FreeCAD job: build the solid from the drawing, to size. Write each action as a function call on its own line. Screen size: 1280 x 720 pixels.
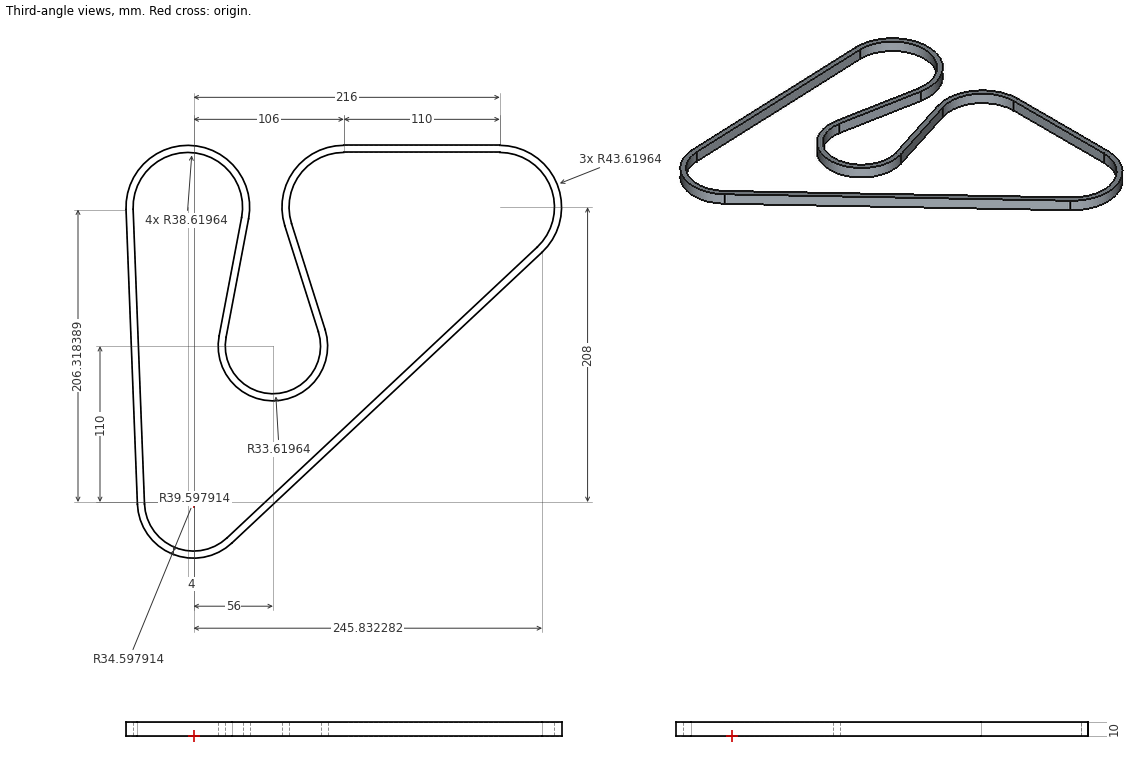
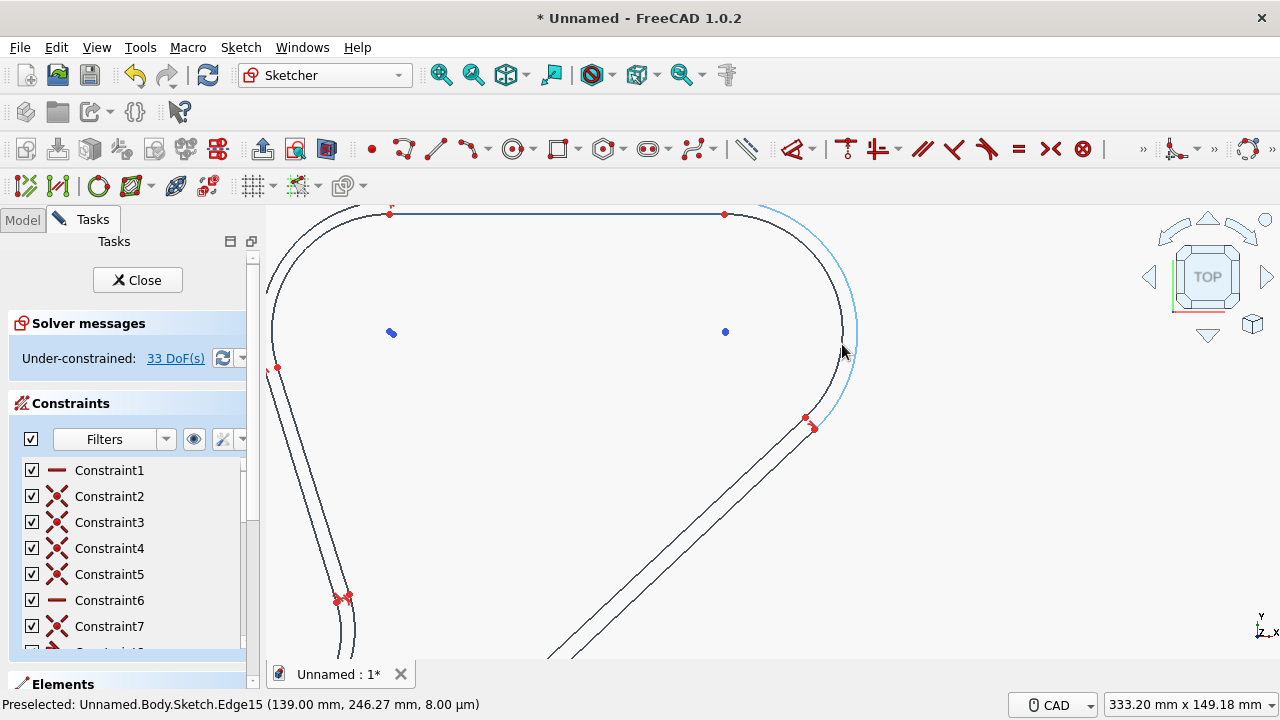
click(842, 343)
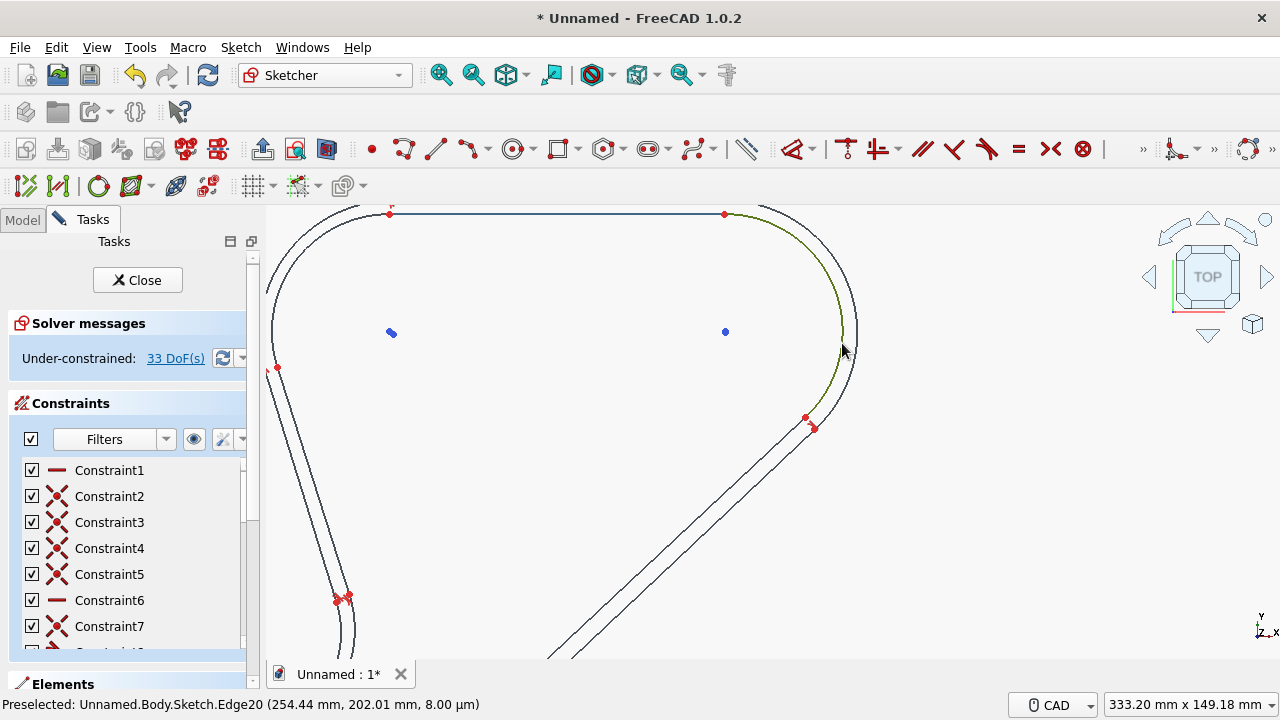
click(988, 150)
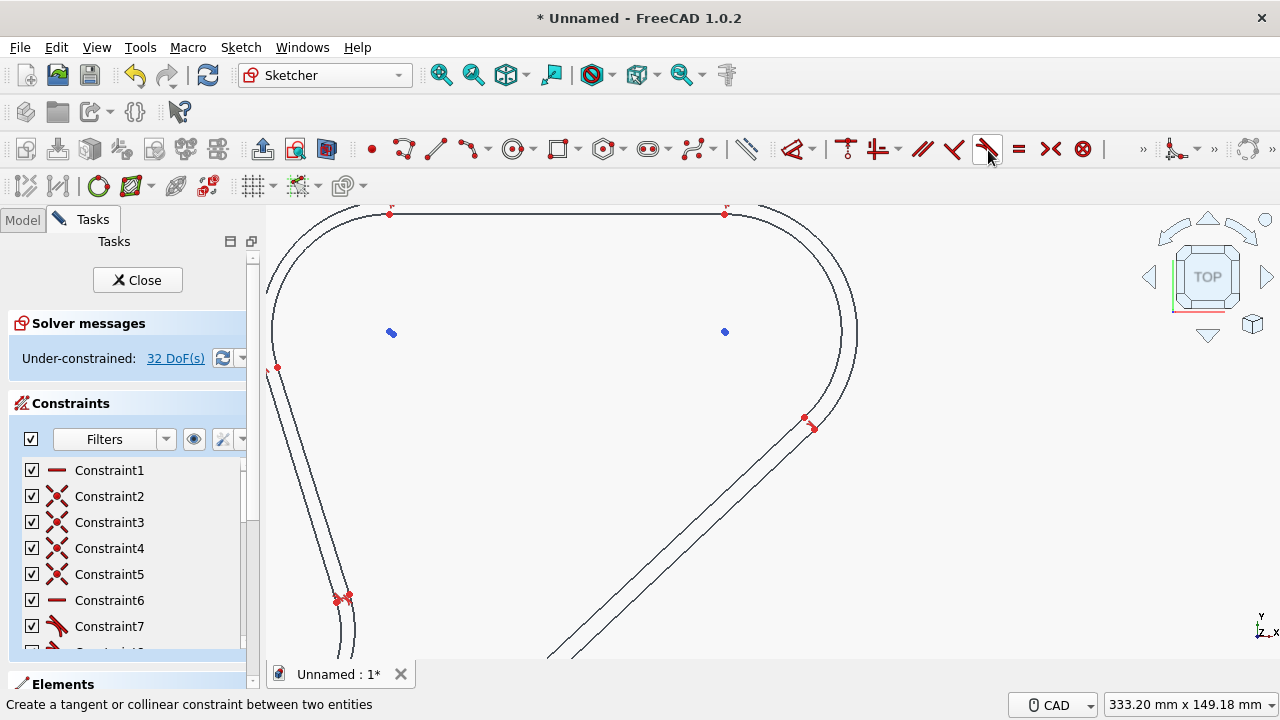
scroll(842, 344, down, 6)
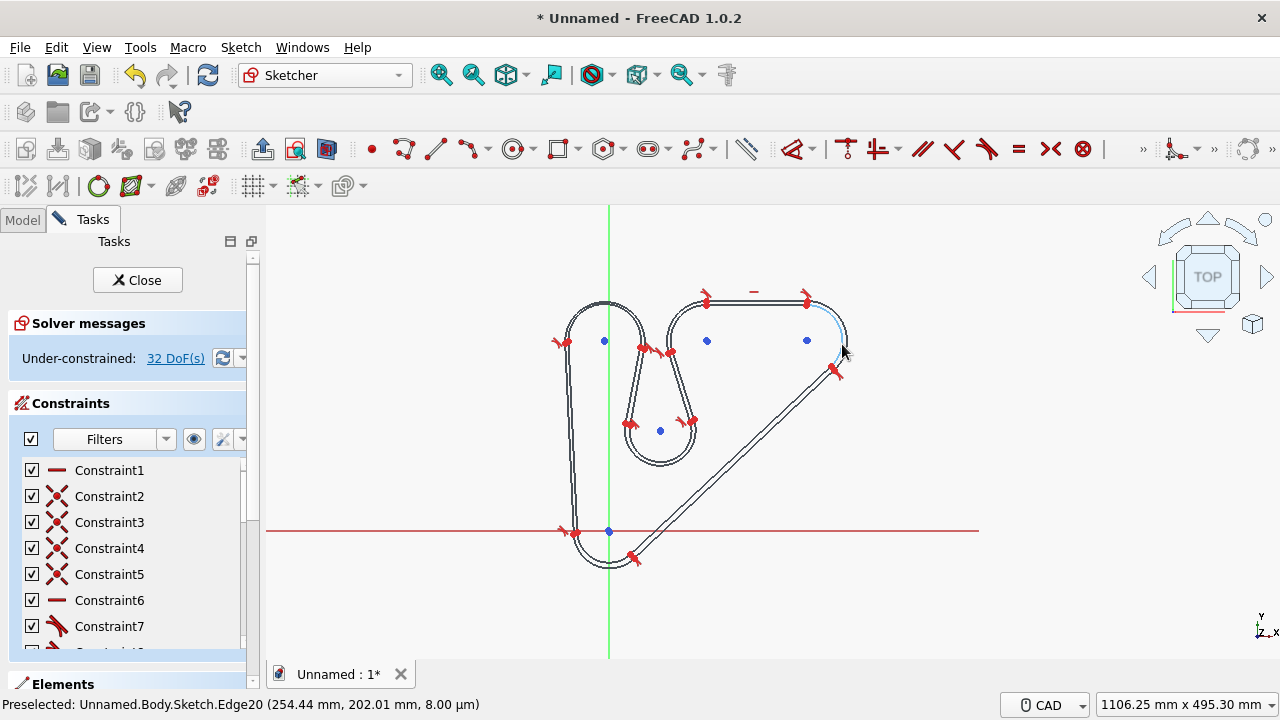
scroll(583, 556, up, 6)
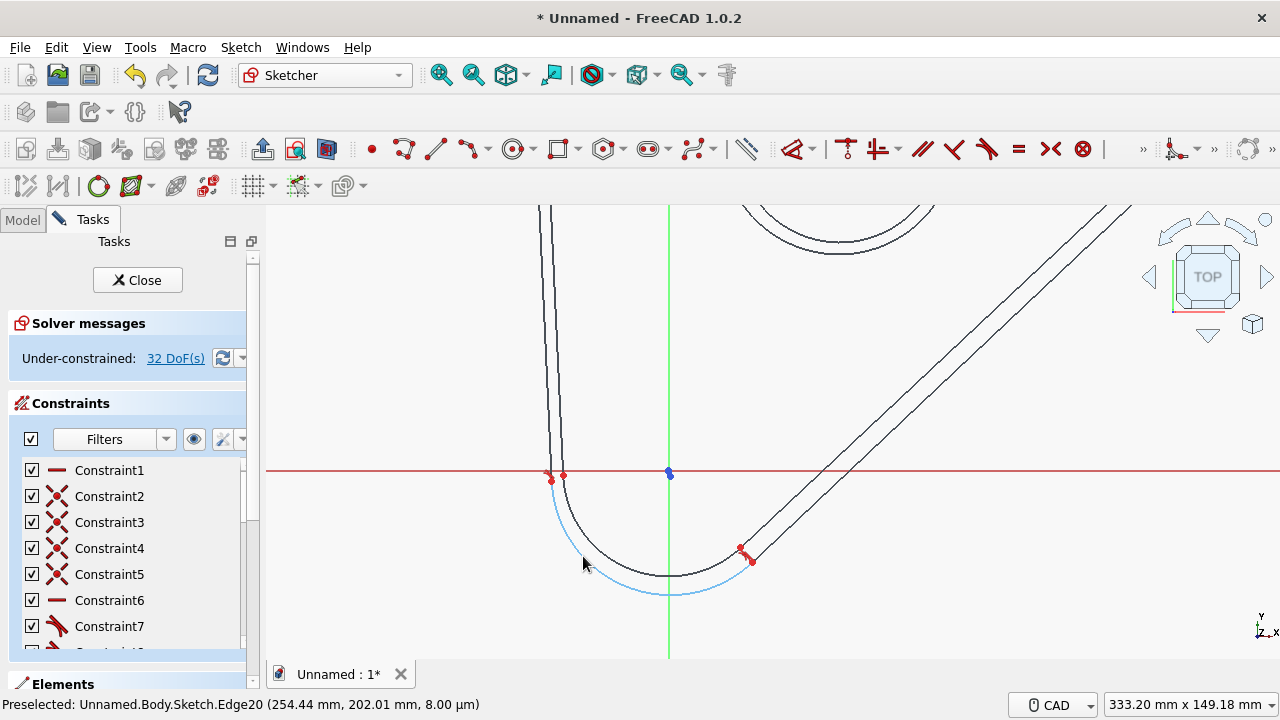
click(582, 555)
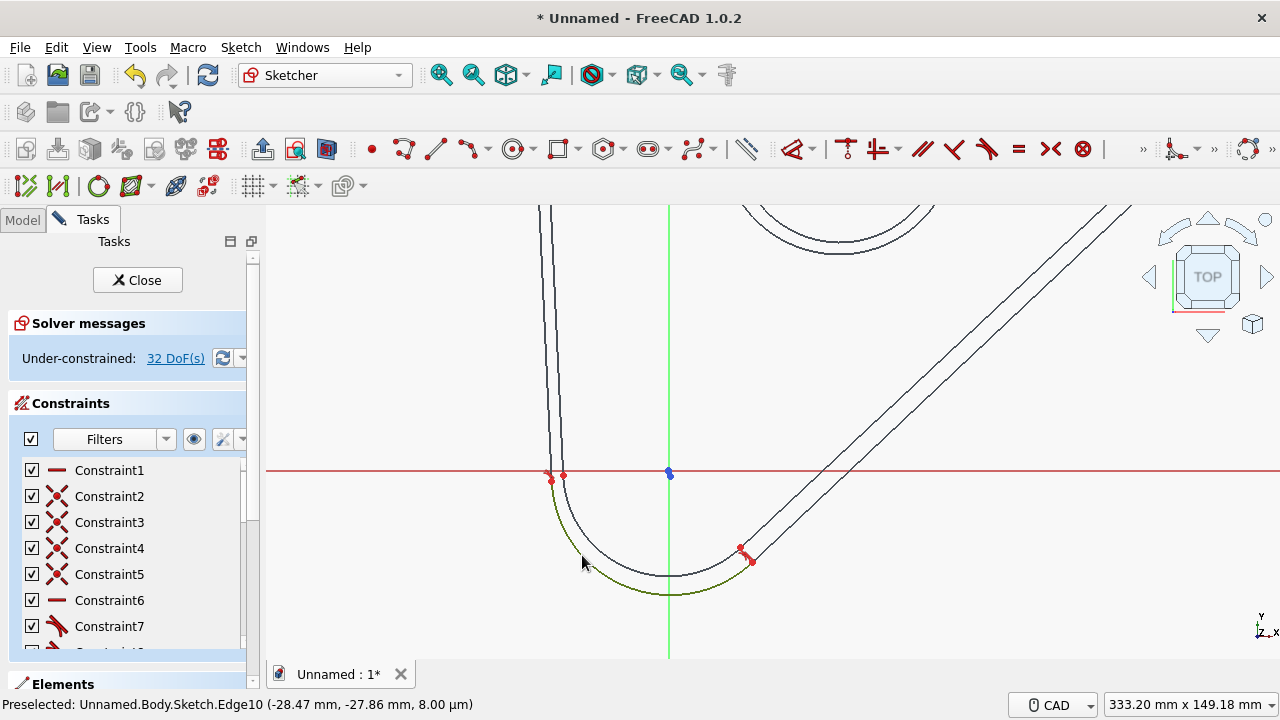
click(590, 541)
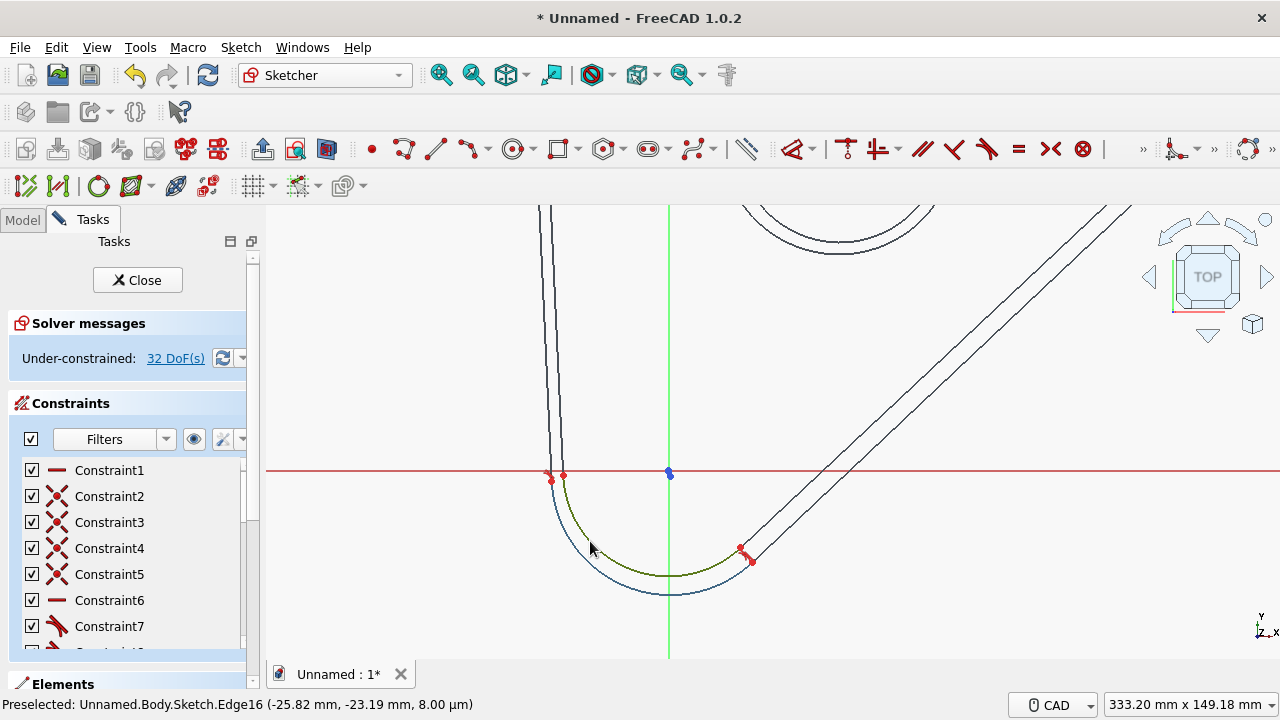
click(846, 150)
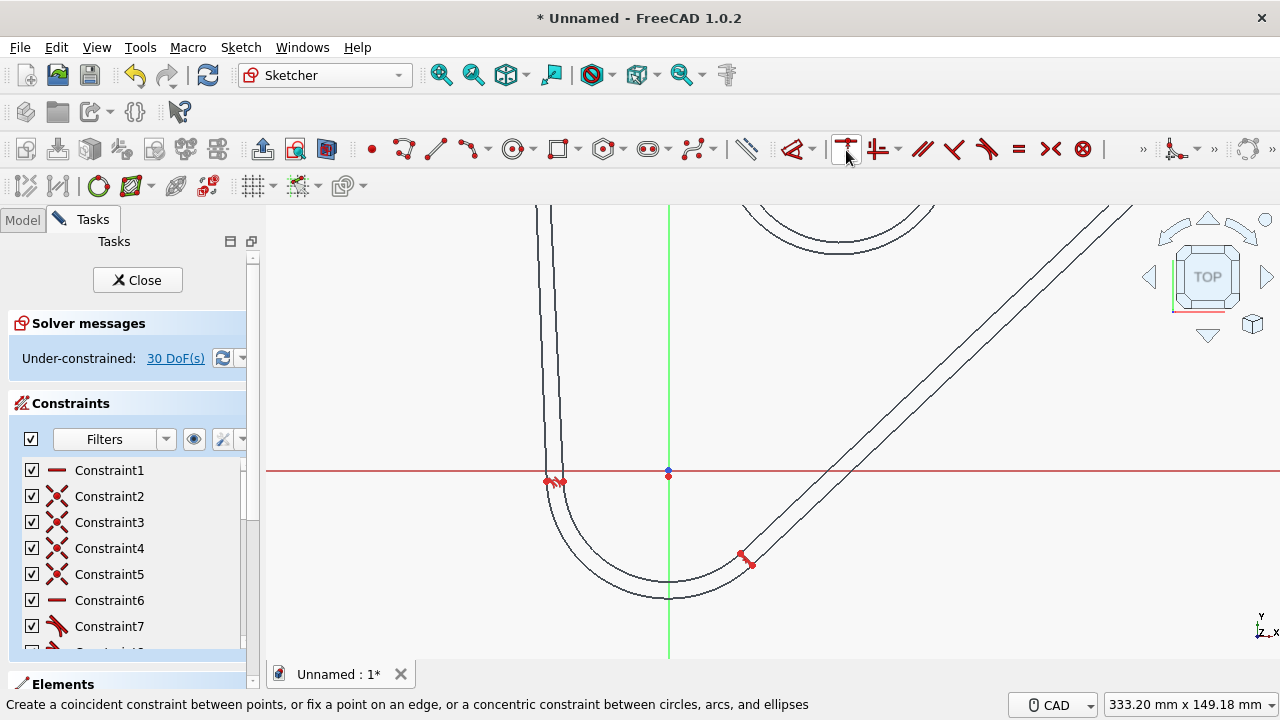
scroll(583, 556, down, 6)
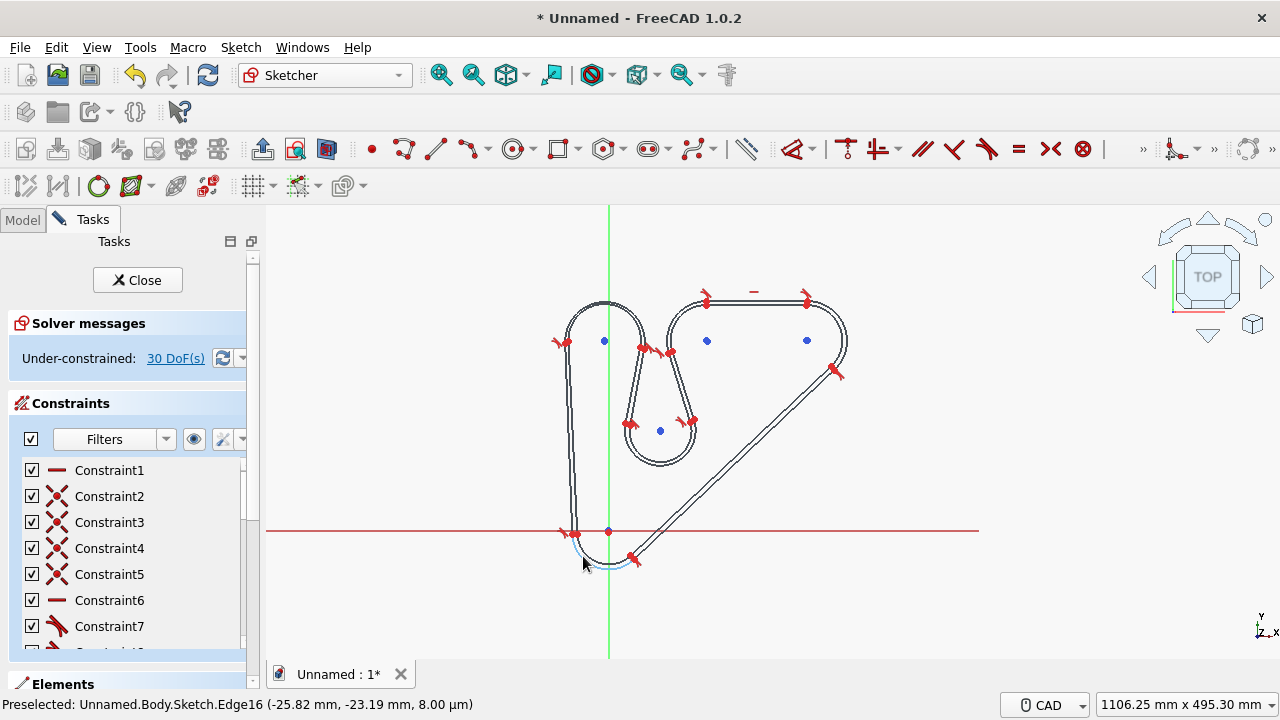
scroll(640, 323, up, 8)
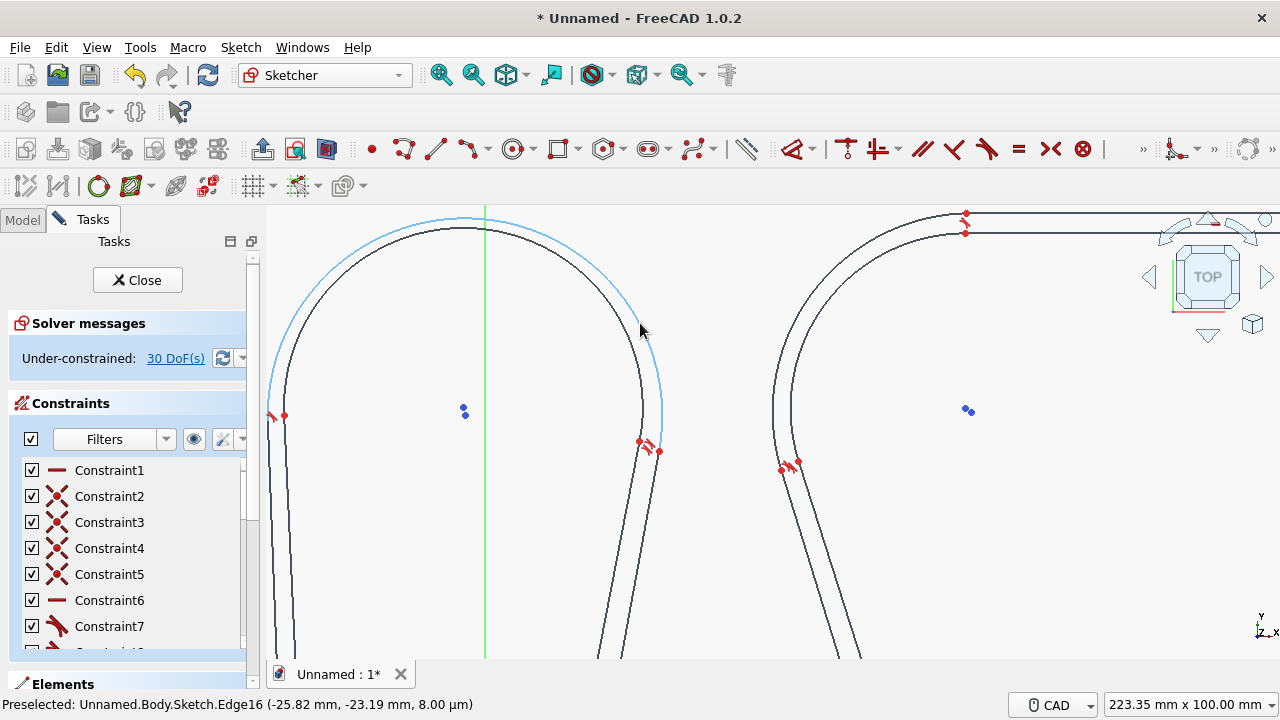
click(639, 323)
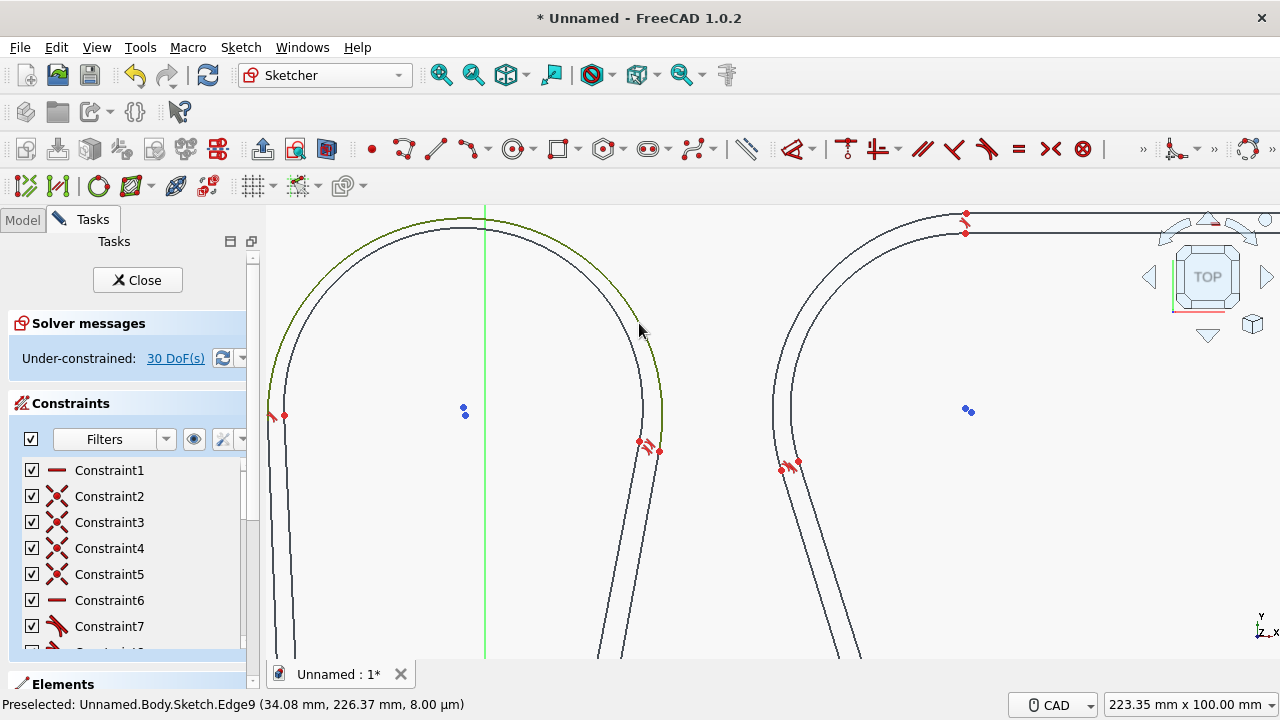
click(585, 276)